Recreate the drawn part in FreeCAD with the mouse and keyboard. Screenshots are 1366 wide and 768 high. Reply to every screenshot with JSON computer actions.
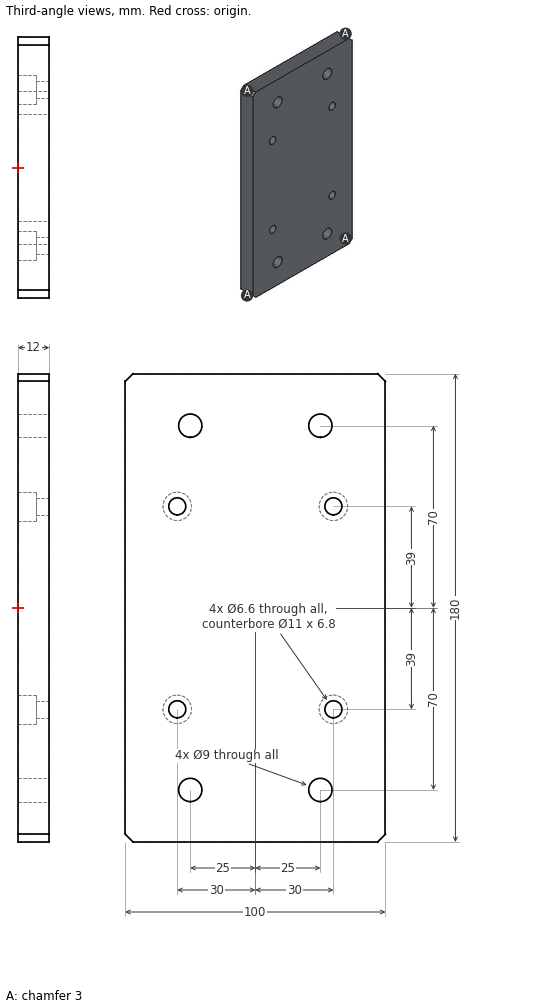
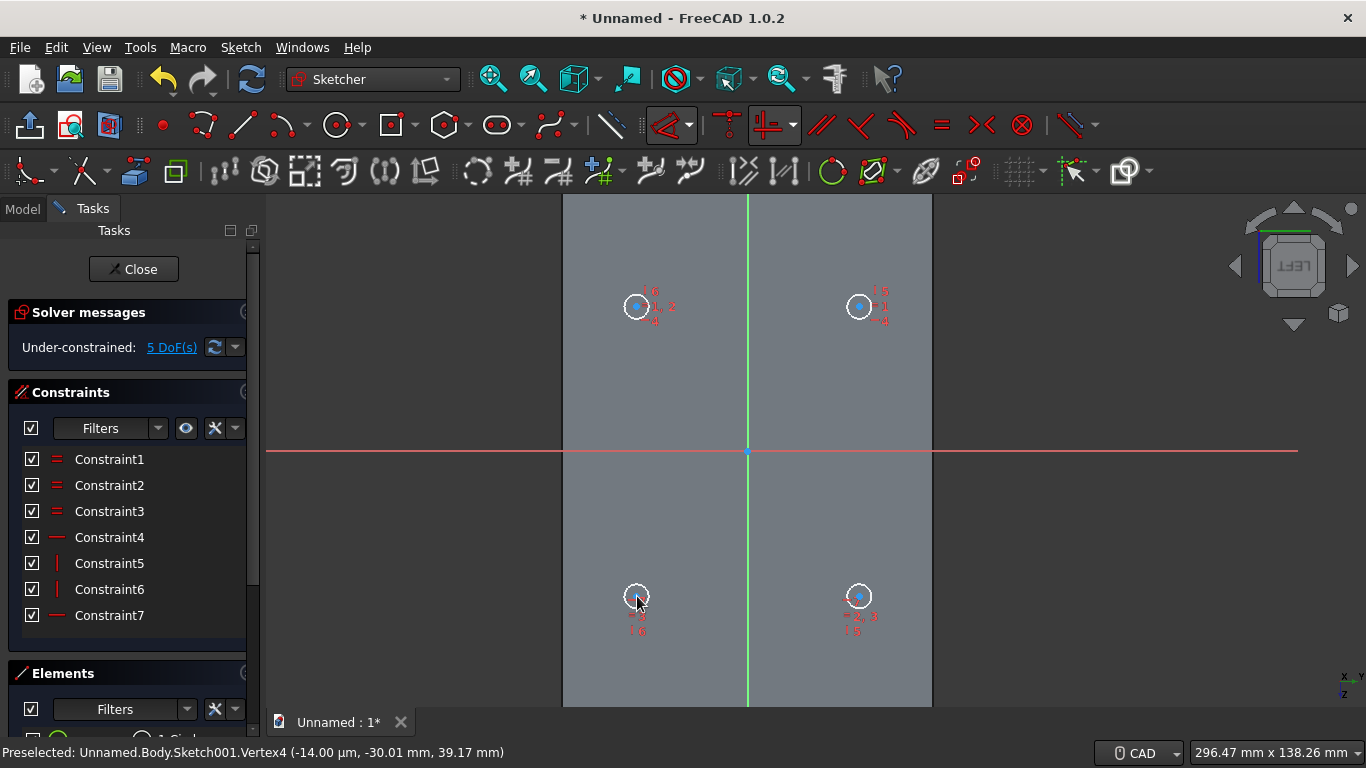
{"action": "scroll", "coordinate": [868, 298], "scroll_direction": "up", "scroll_amount": 3}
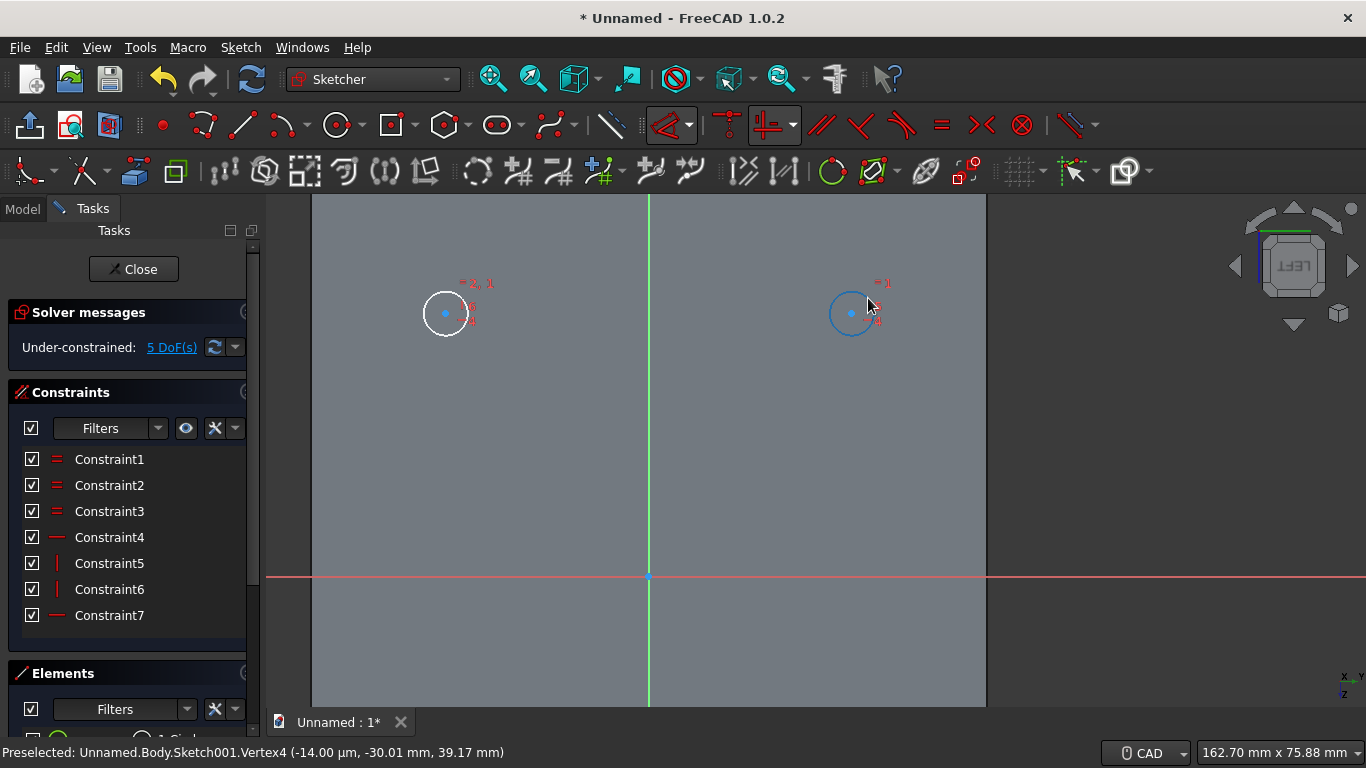
{"action": "left_click", "coordinate": [836, 298]}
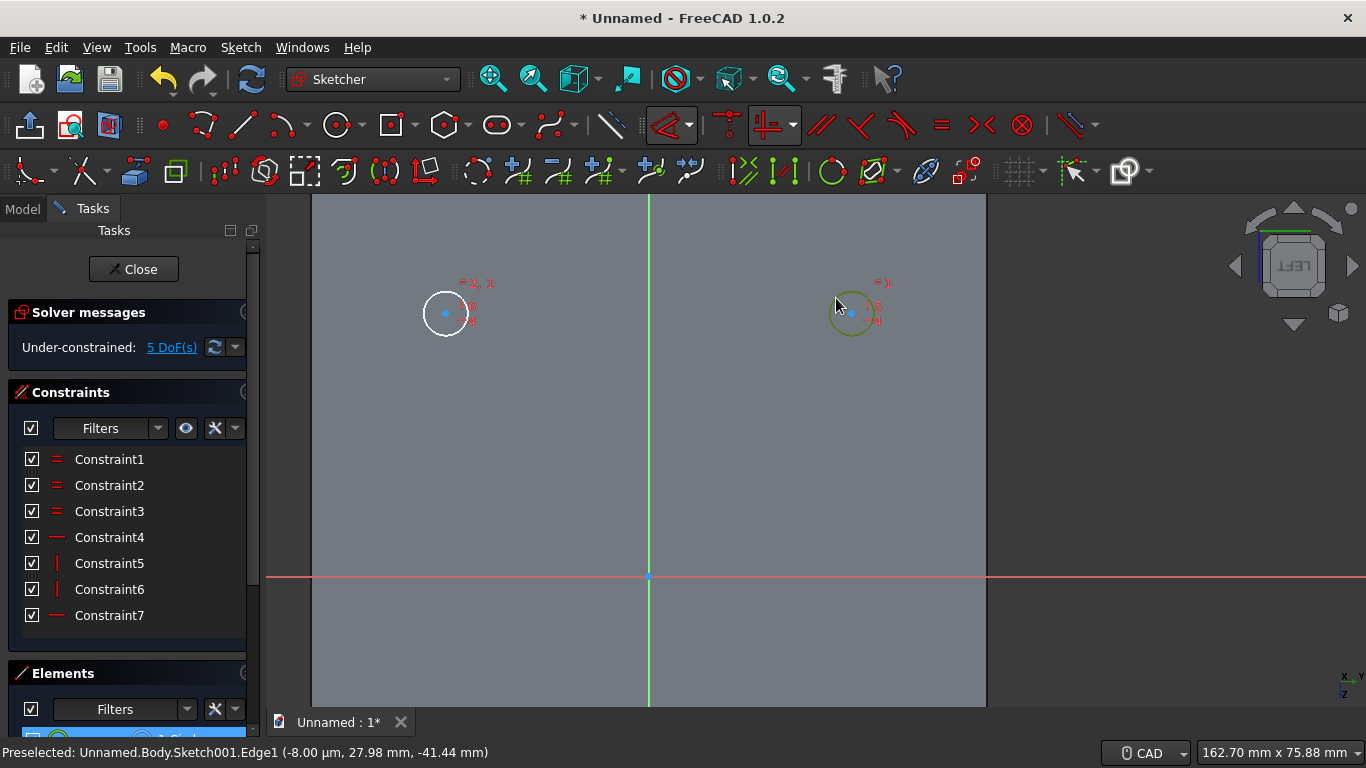
{"action": "key", "text": "k o"}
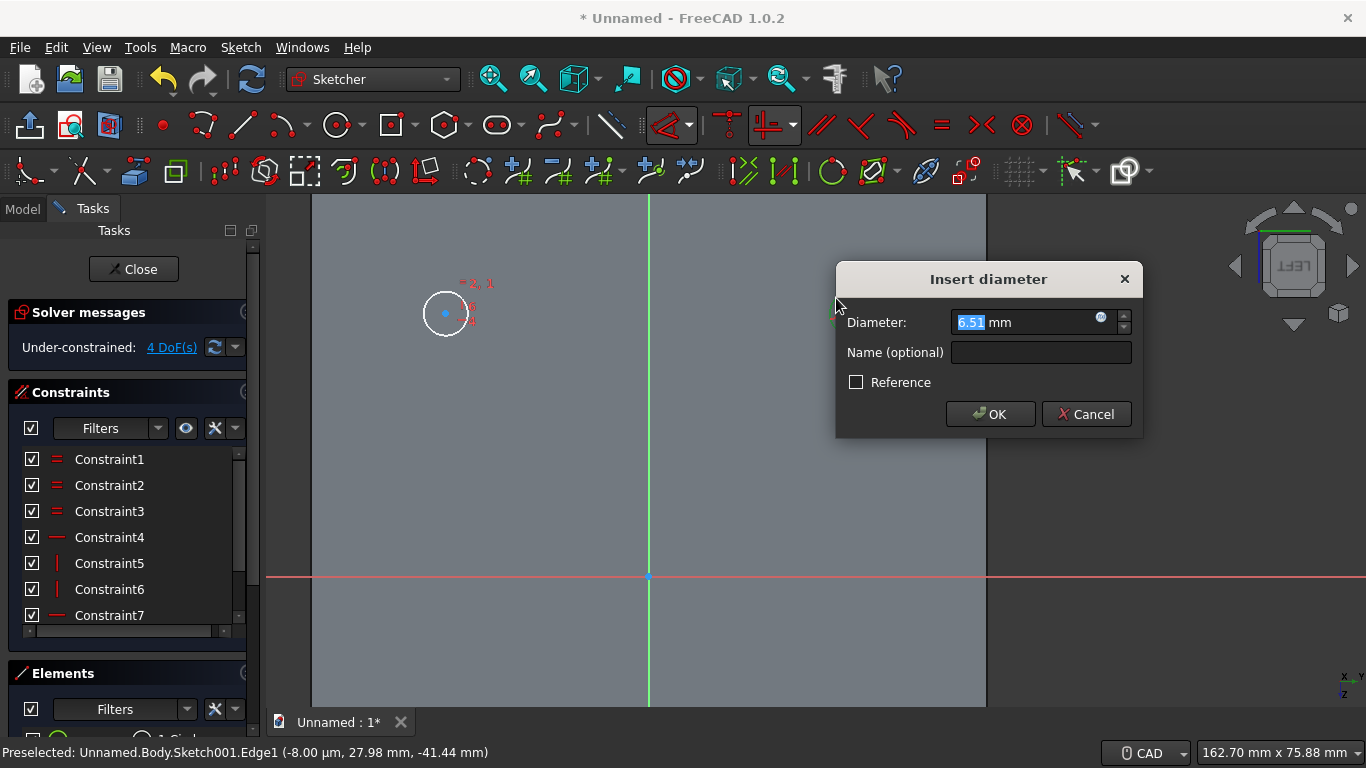
{"action": "type", "text": "6.6"}
{"action": "key", "text": "Return"}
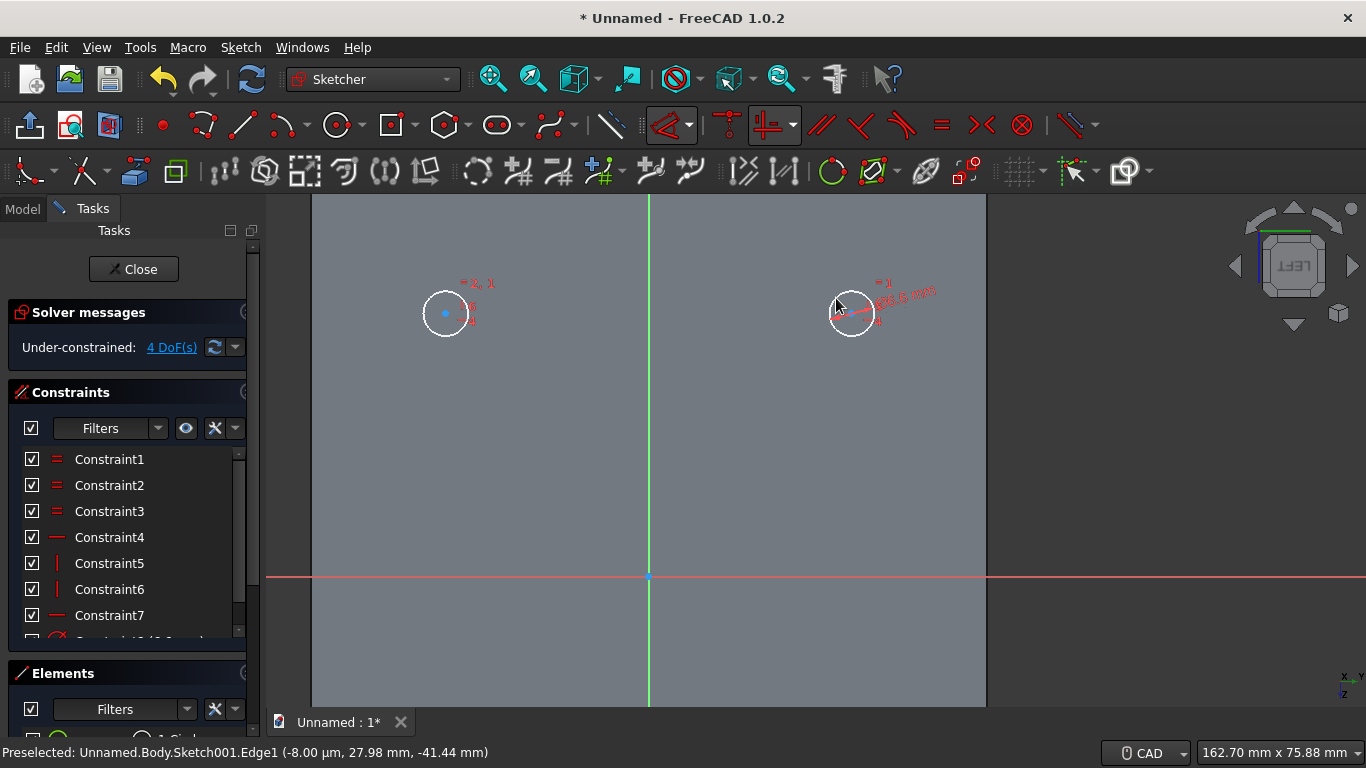
{"action": "left_click", "coordinate": [852, 314]}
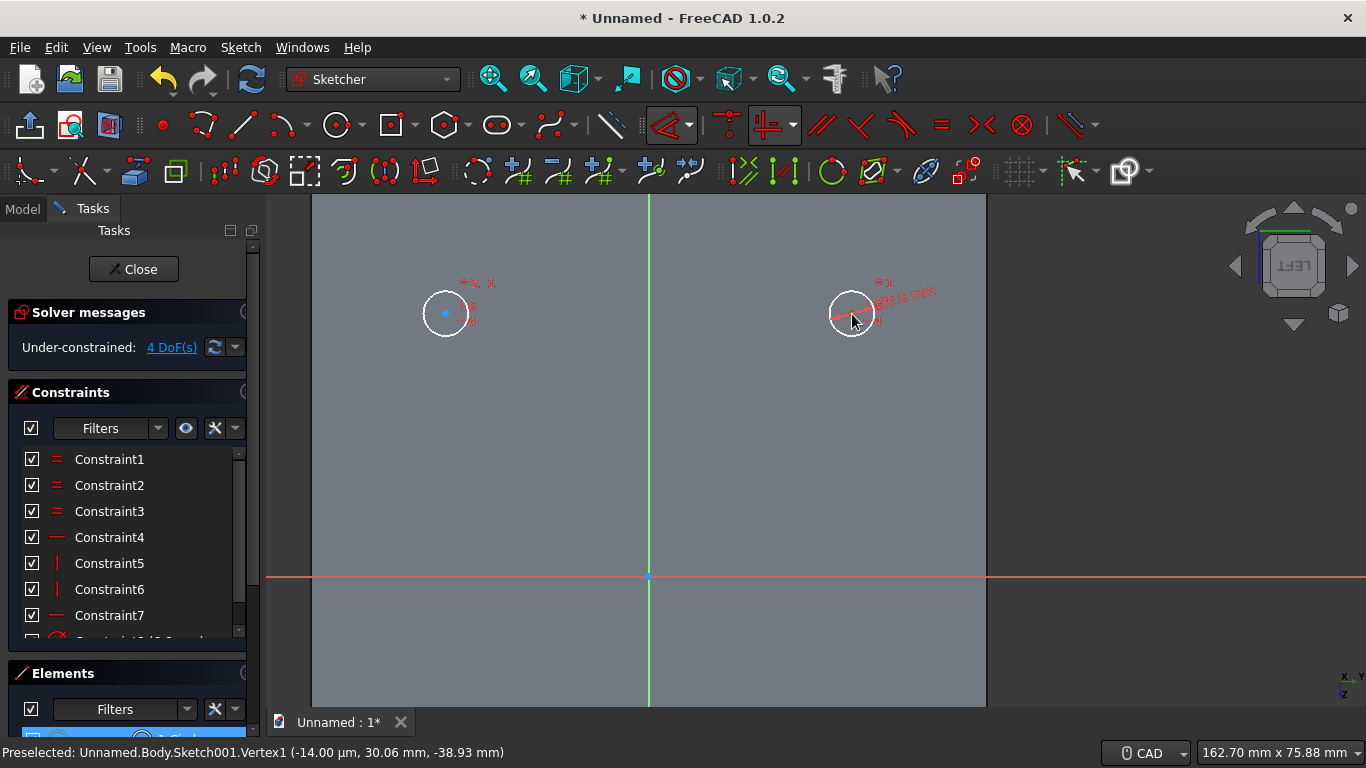
{"action": "key", "text": "l"}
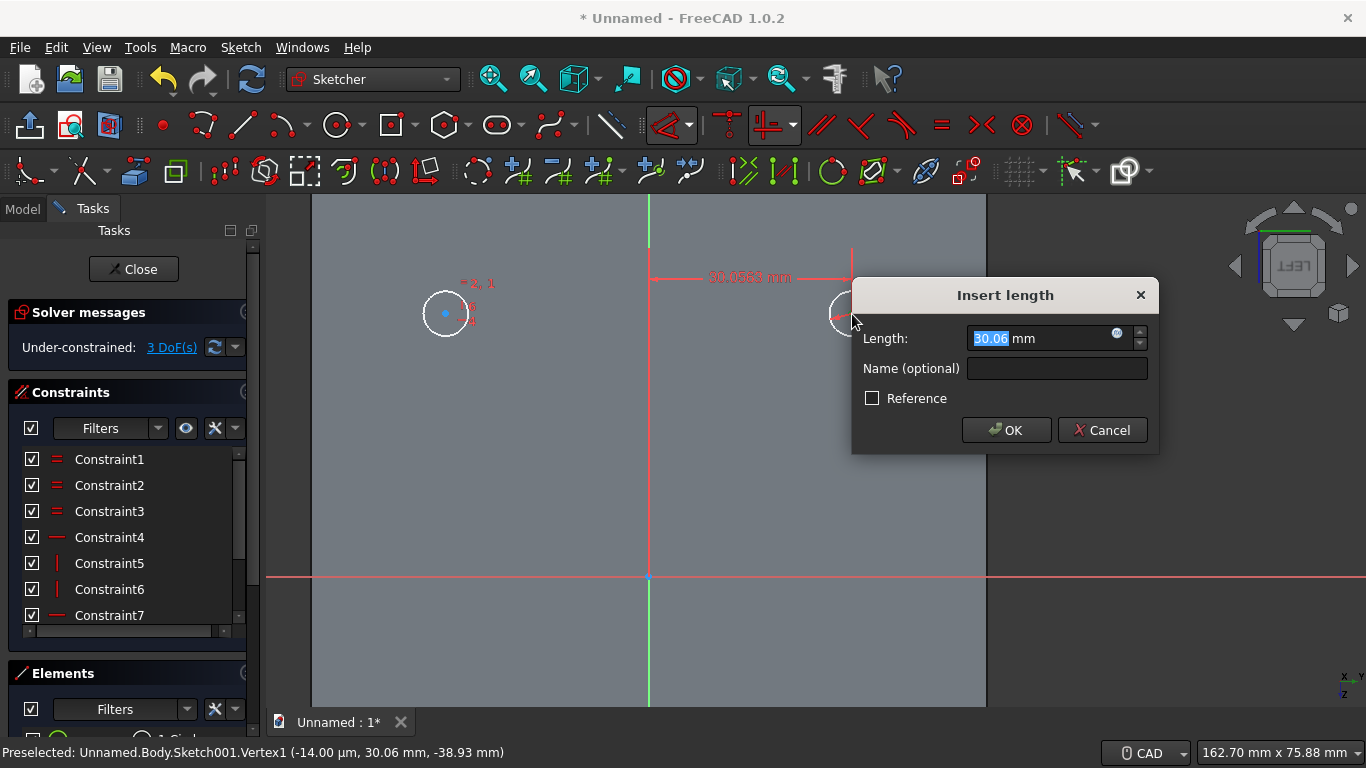
{"action": "type", "text": "30"}
{"action": "key", "text": "Return"}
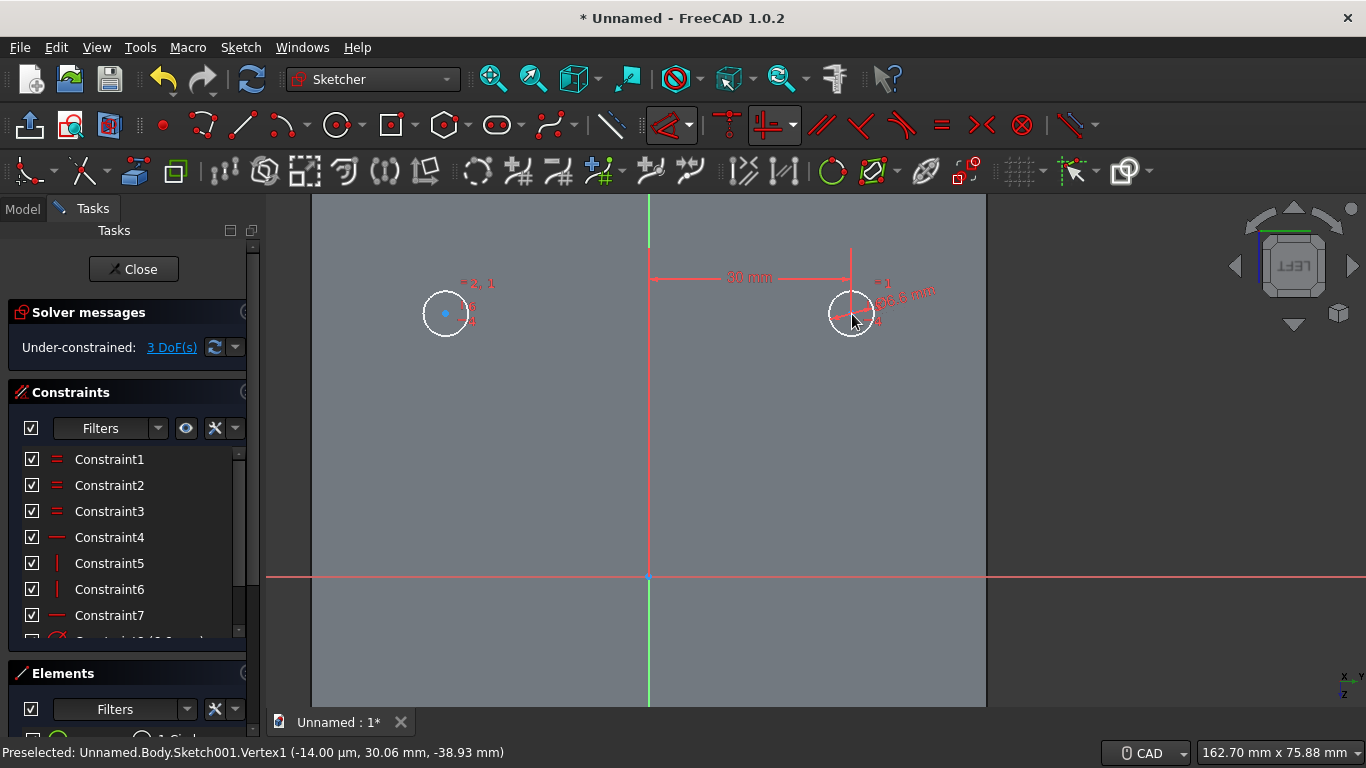
{"action": "left_click", "coordinate": [851, 314]}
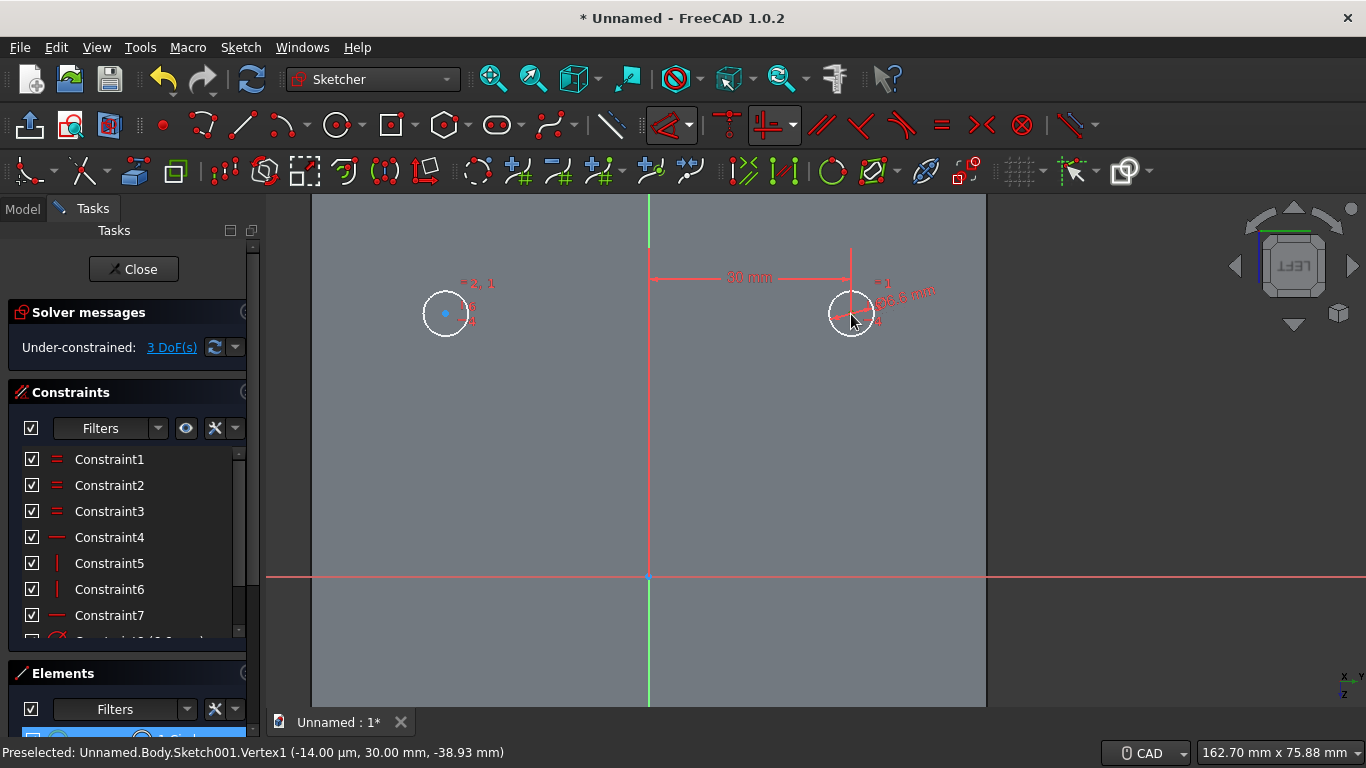
{"action": "key", "text": "i"}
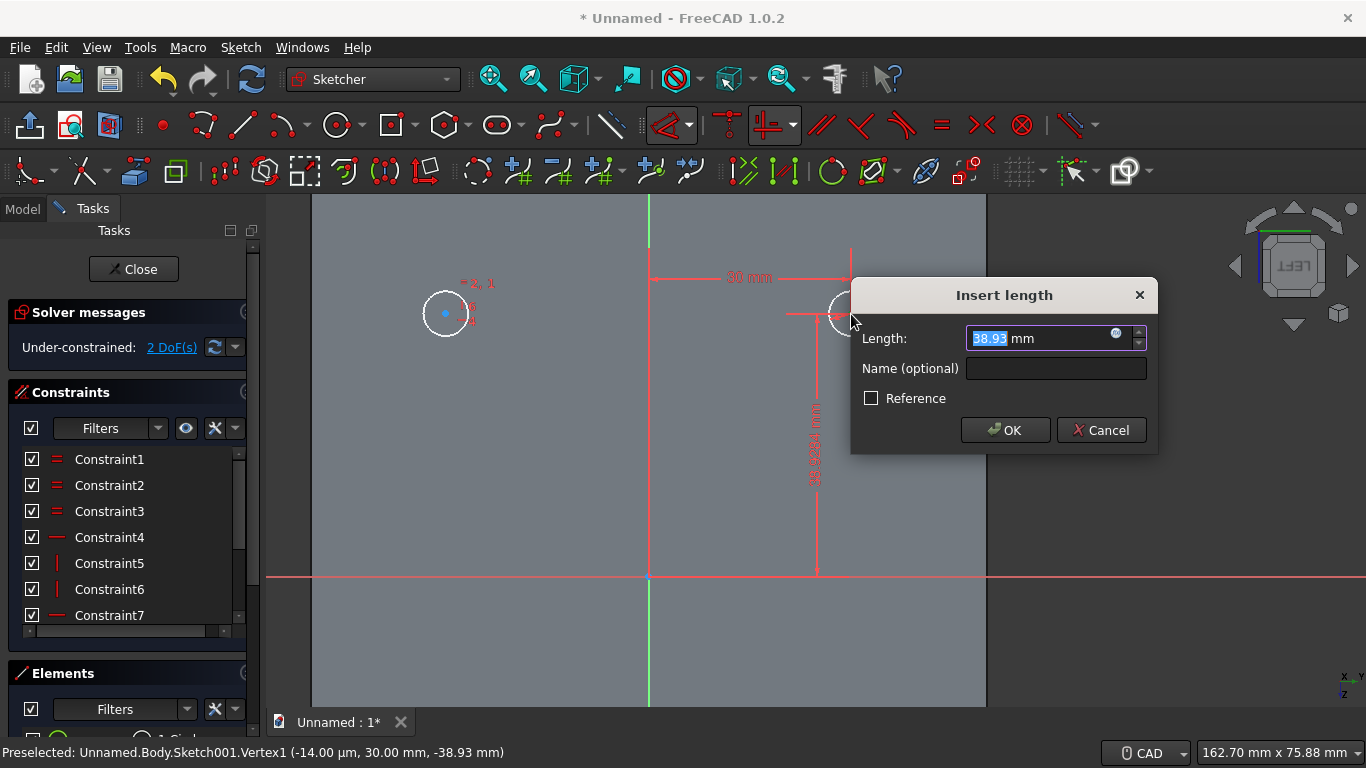
{"action": "type", "text": "39"}
{"action": "key", "text": "Return"}